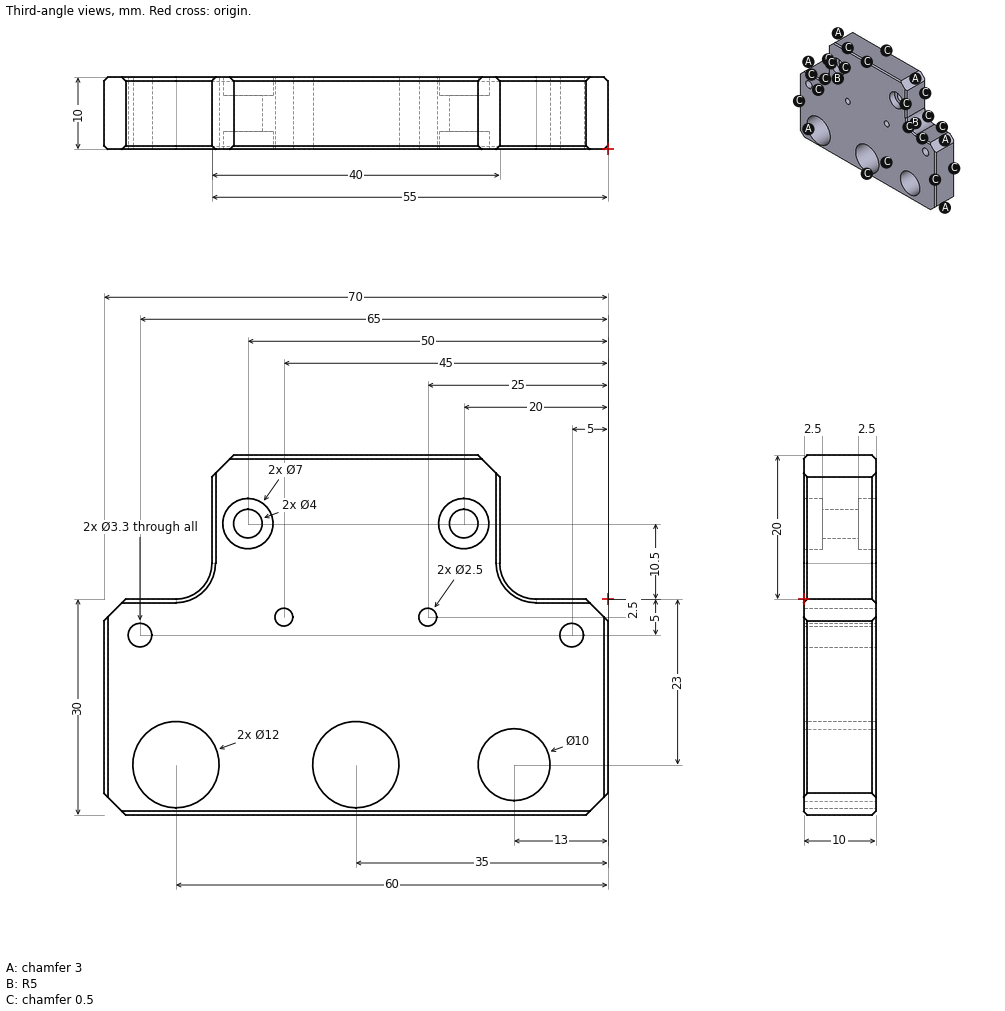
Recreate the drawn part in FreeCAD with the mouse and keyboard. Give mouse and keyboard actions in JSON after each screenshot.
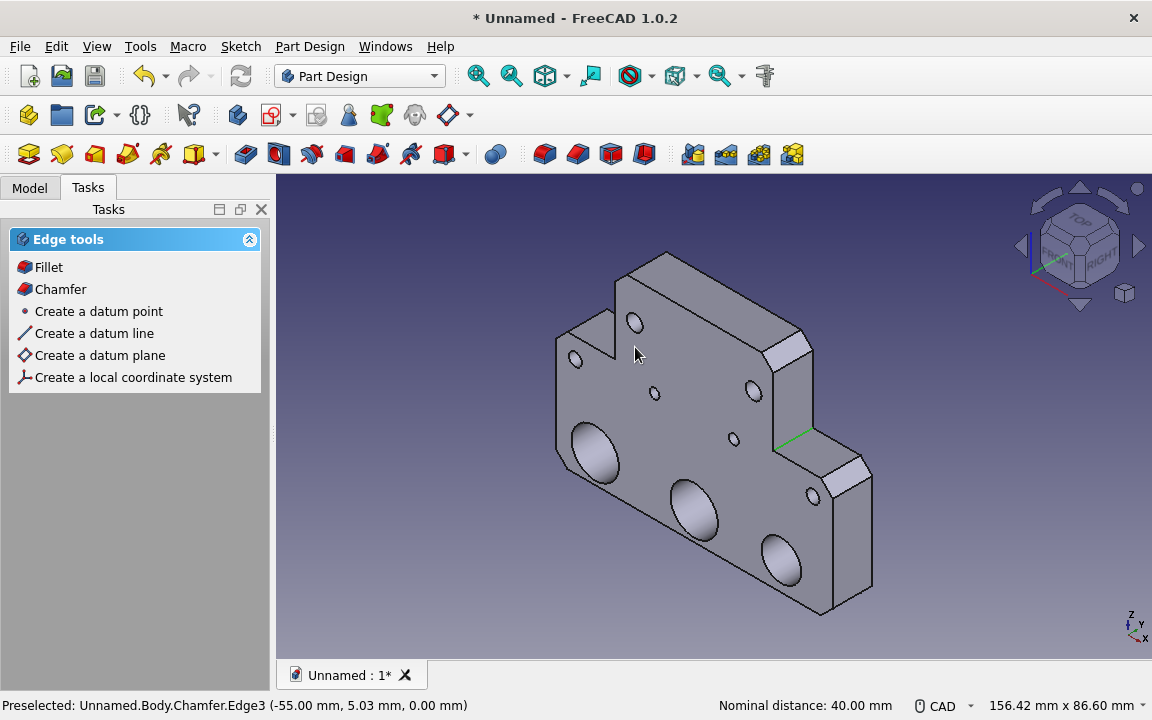
{"action": "left_click", "coordinate": [545, 154]}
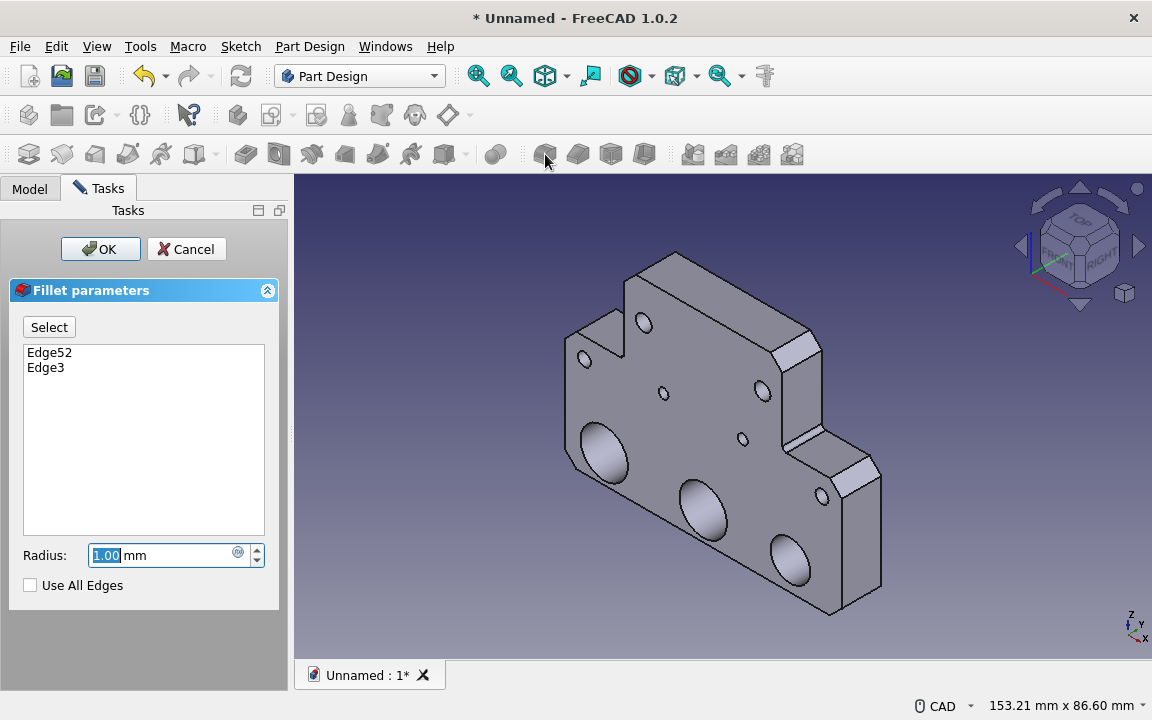
{"action": "type", "text": "5"}
{"action": "key", "text": "Tab"}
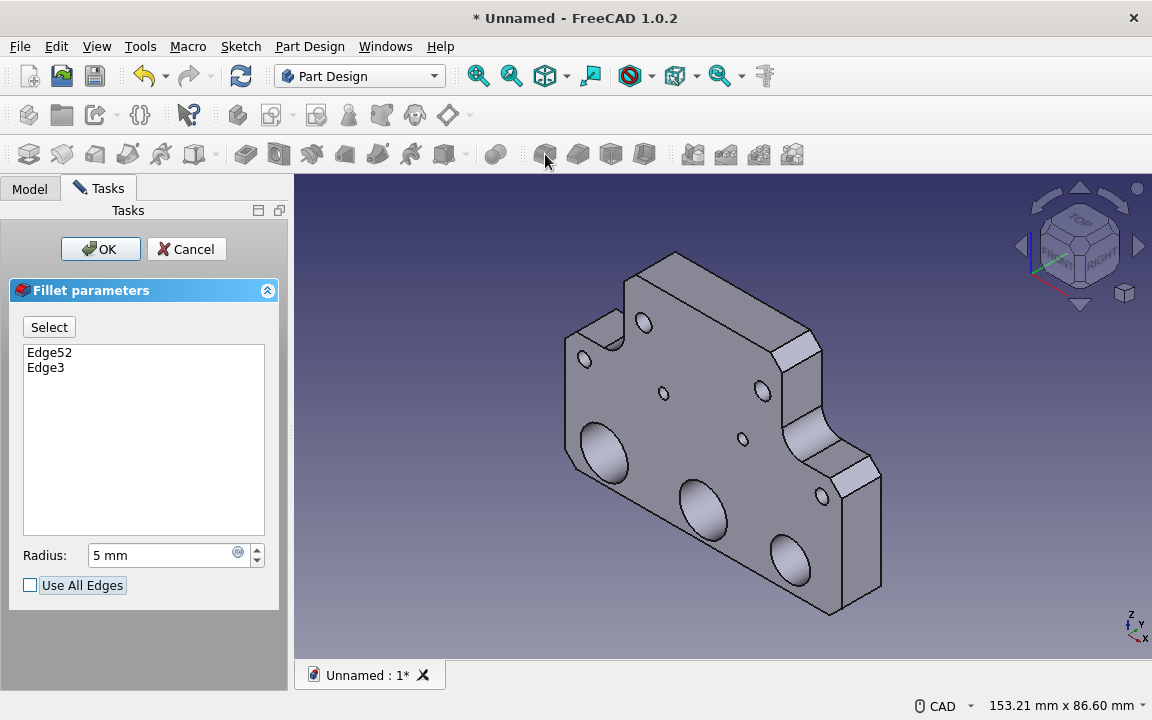
{"action": "left_click", "coordinate": [101, 249]}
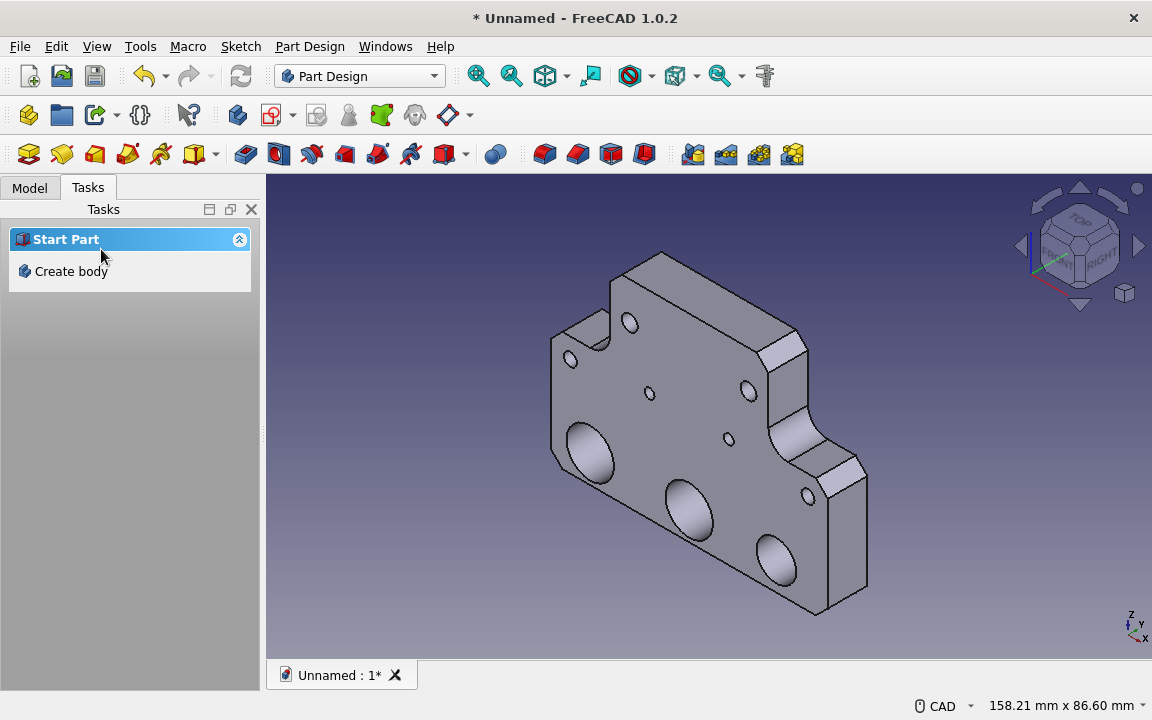
{"action": "left_click", "coordinate": [802, 469]}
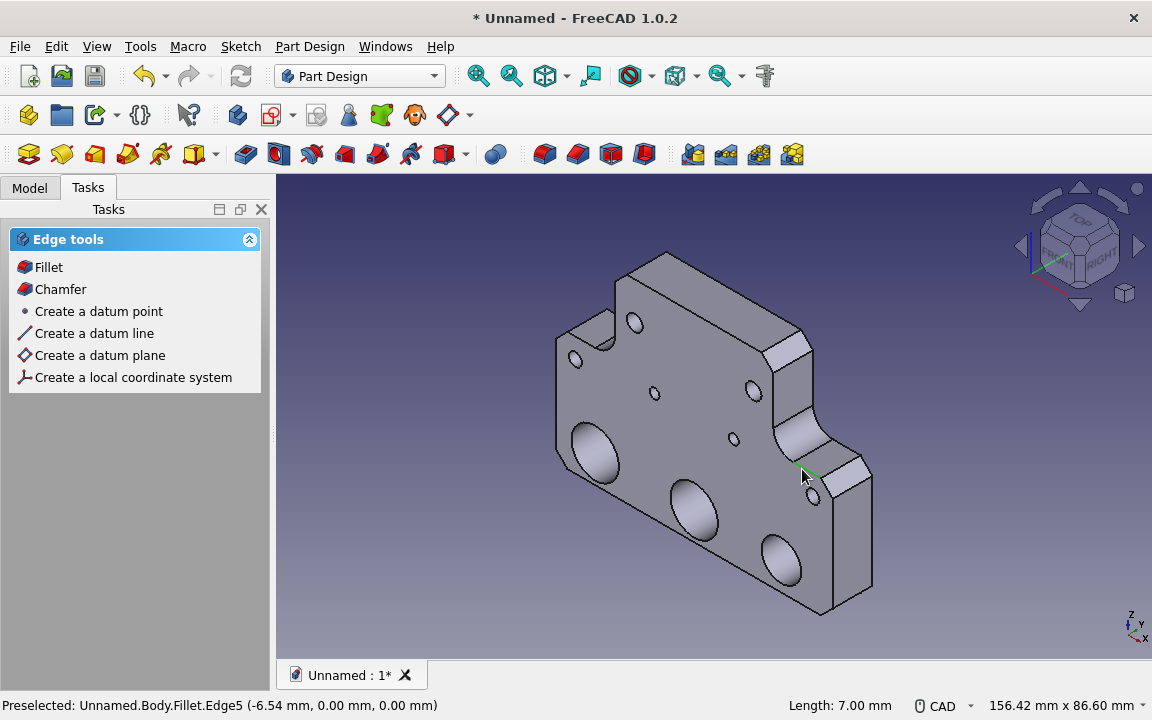
{"action": "left_click", "coordinate": [779, 446], "text": "ctrl"}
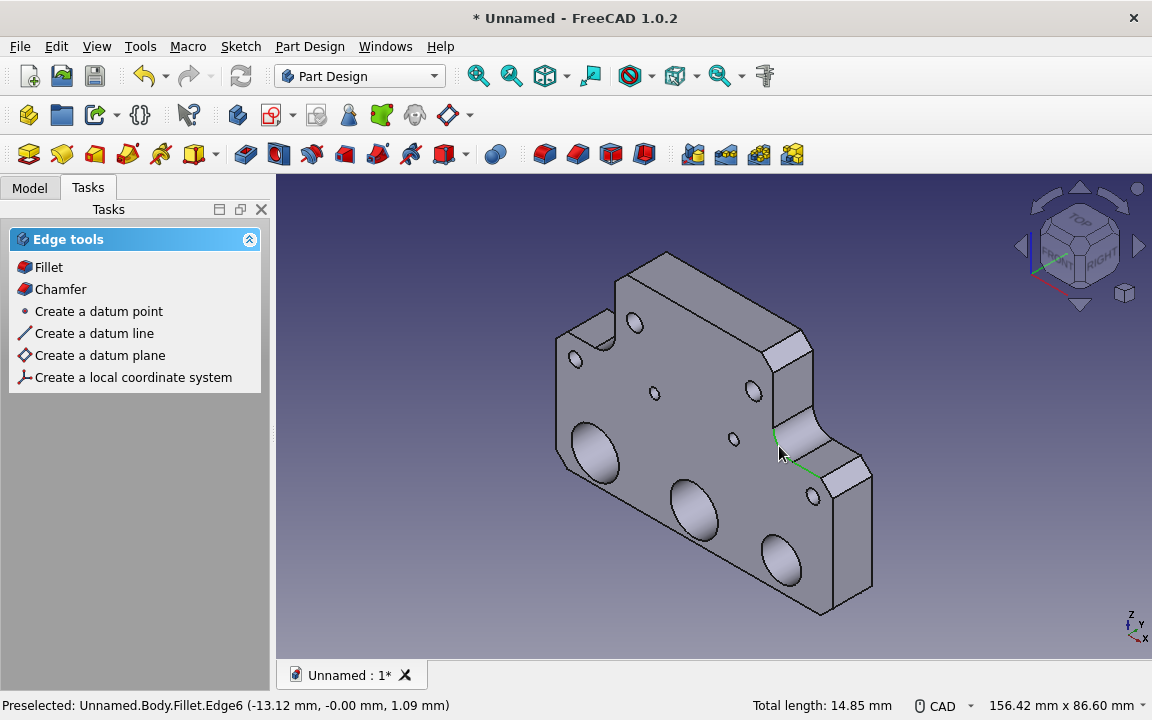
{"action": "left_click", "coordinate": [607, 349], "text": "ctrl"}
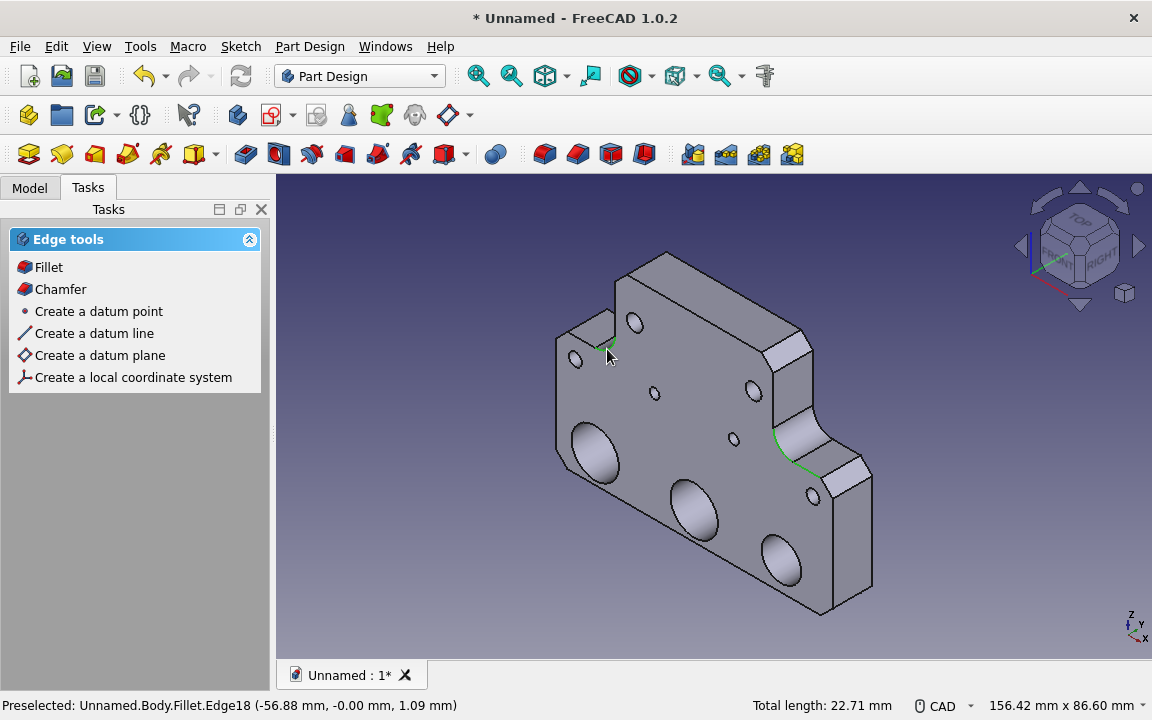
{"action": "left_click", "coordinate": [833, 553], "text": "ctrl"}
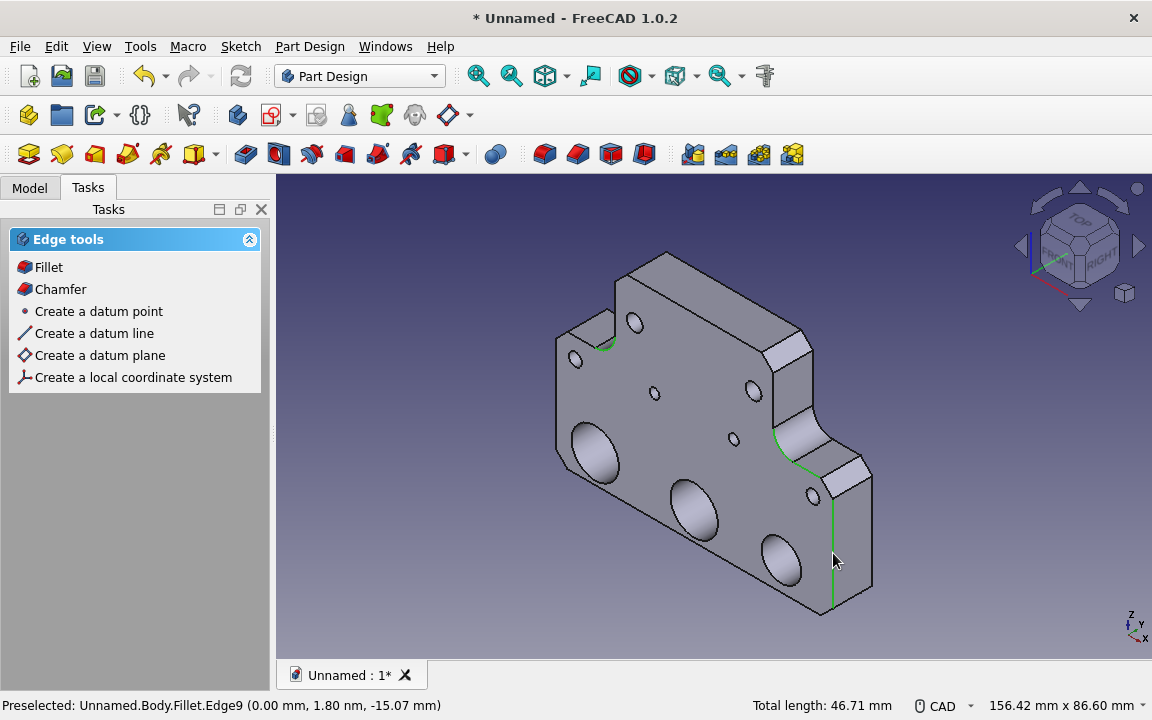
{"action": "left_click", "coordinate": [773, 399], "text": "ctrl"}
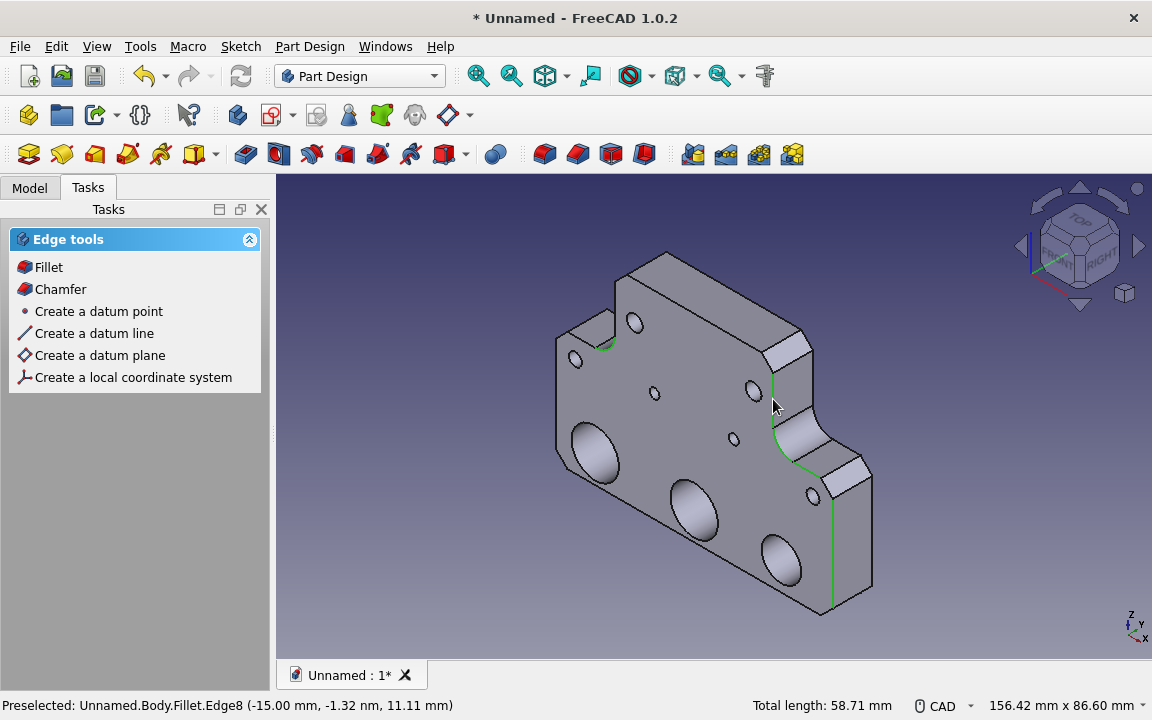
{"action": "left_click", "coordinate": [694, 313], "text": "ctrl"}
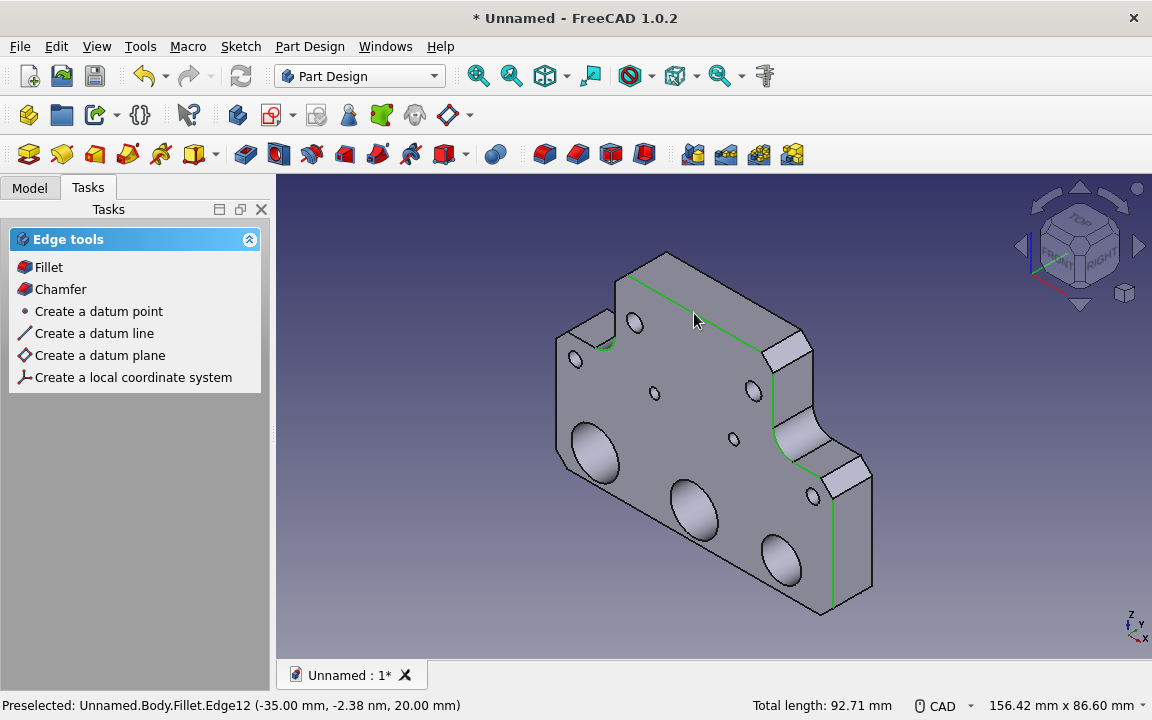
{"action": "left_click", "coordinate": [581, 339], "text": "ctrl"}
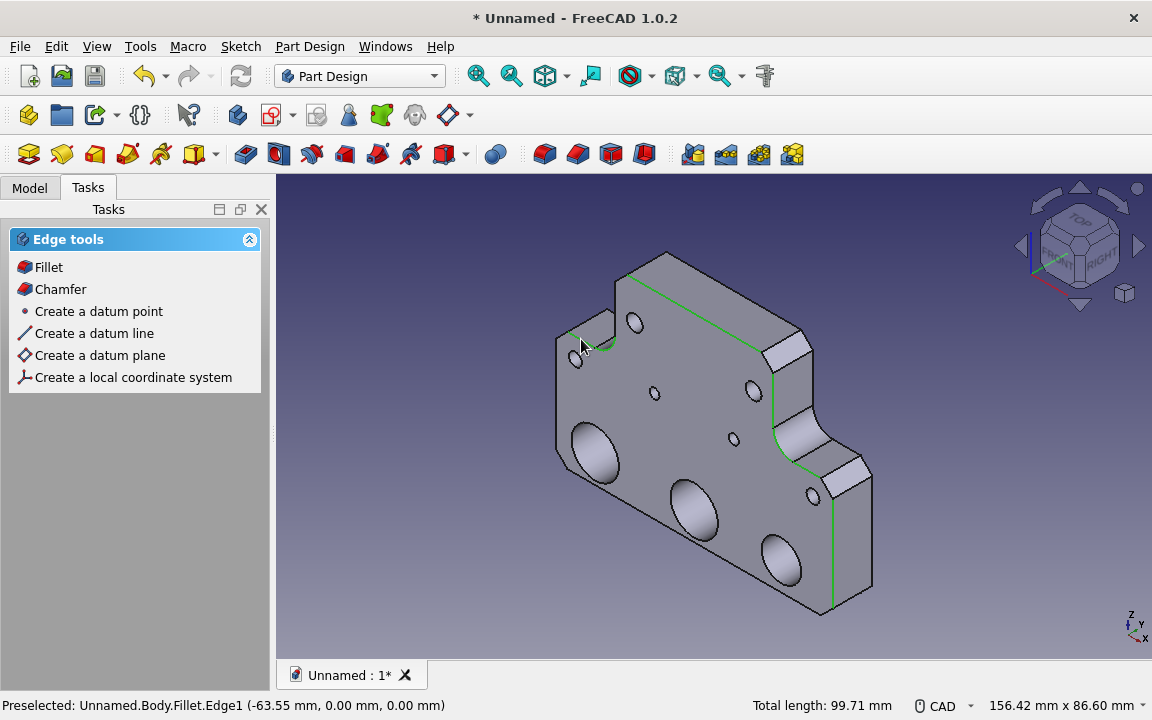
{"action": "key", "text": "2"}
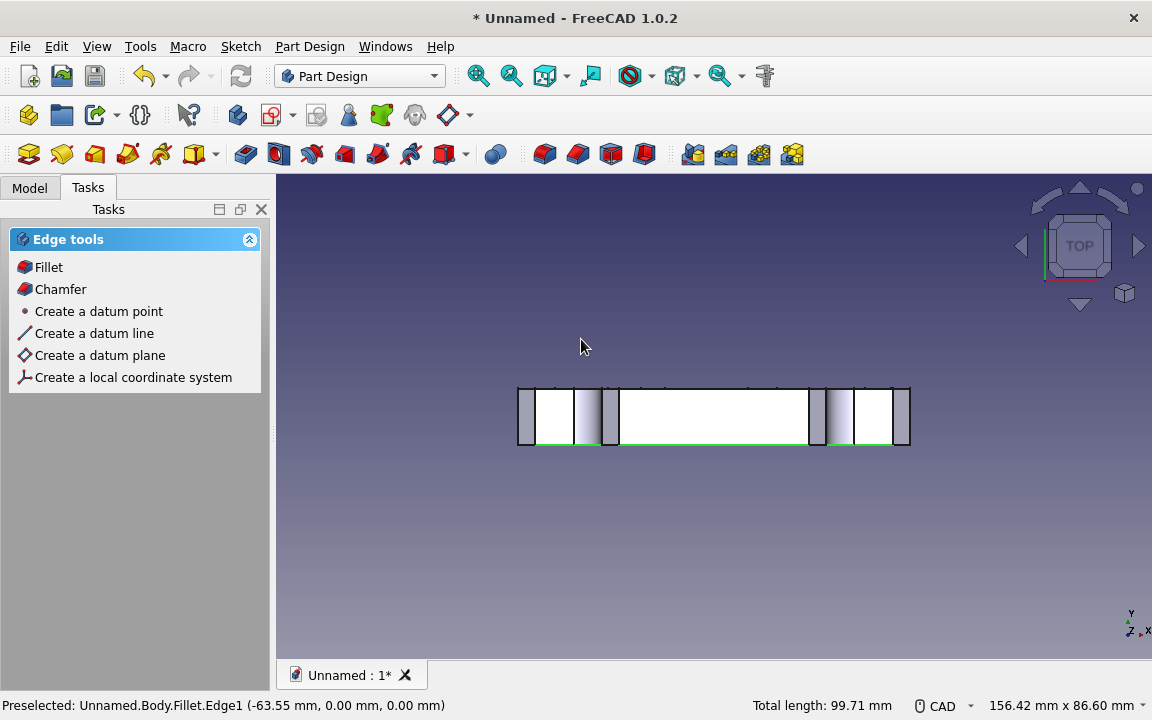
{"action": "left_click", "coordinate": [479, 76]}